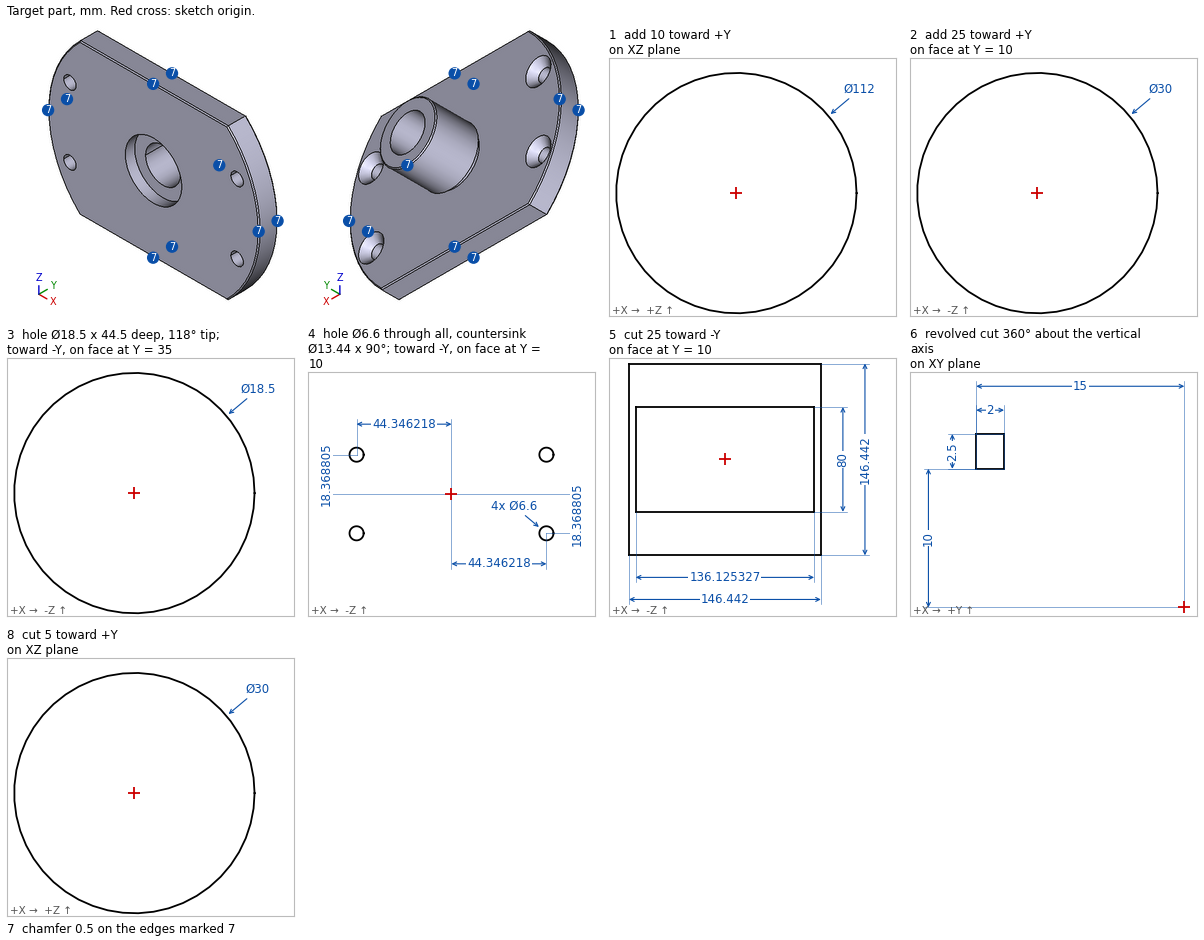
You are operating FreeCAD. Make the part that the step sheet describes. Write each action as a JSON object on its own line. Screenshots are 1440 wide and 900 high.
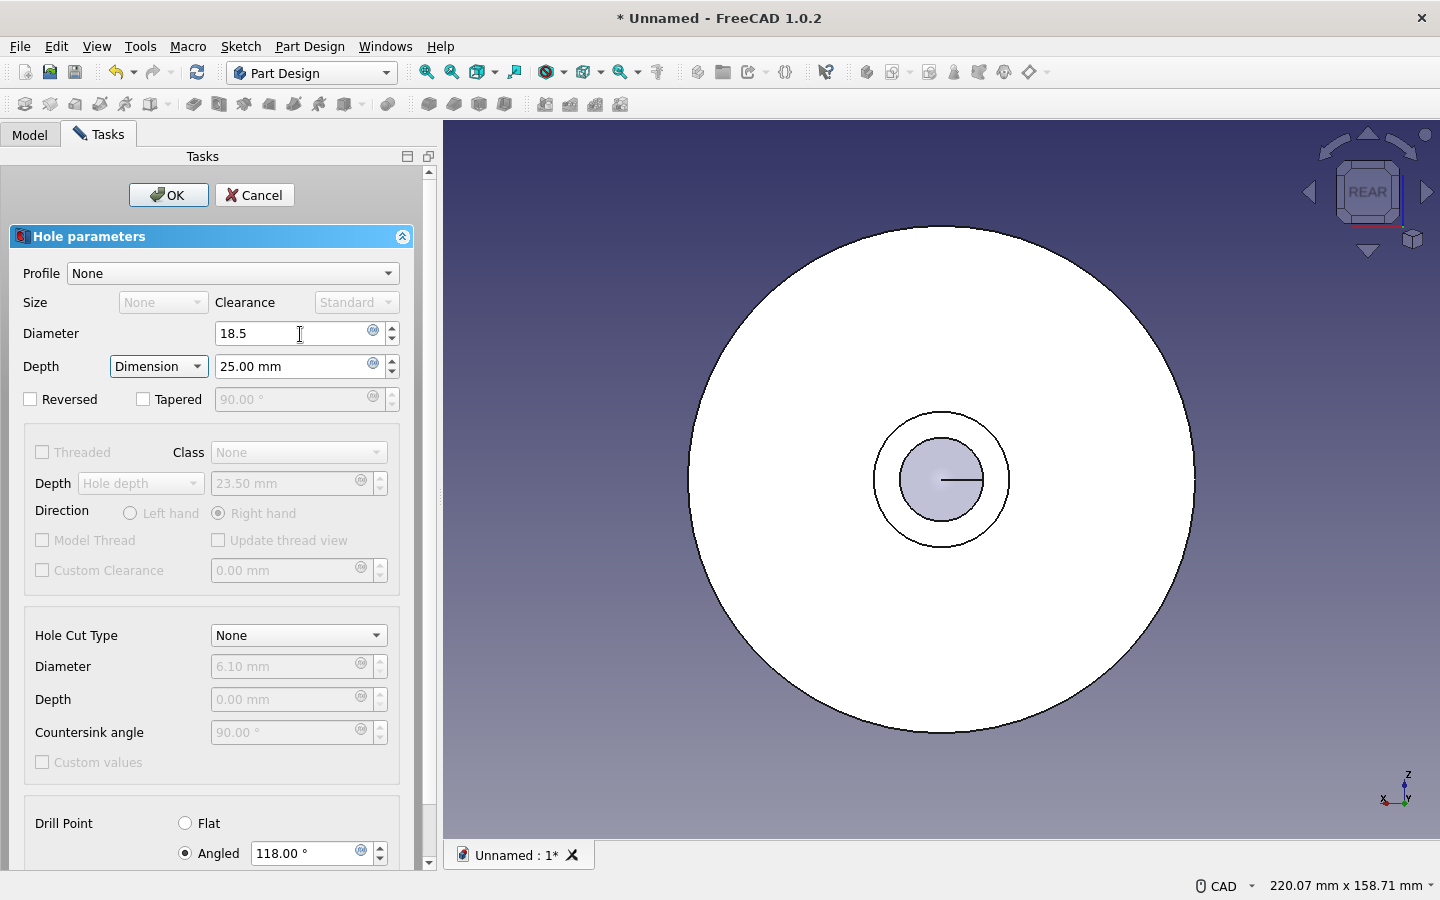
{"action": "triple_click", "coordinate": [300, 366]}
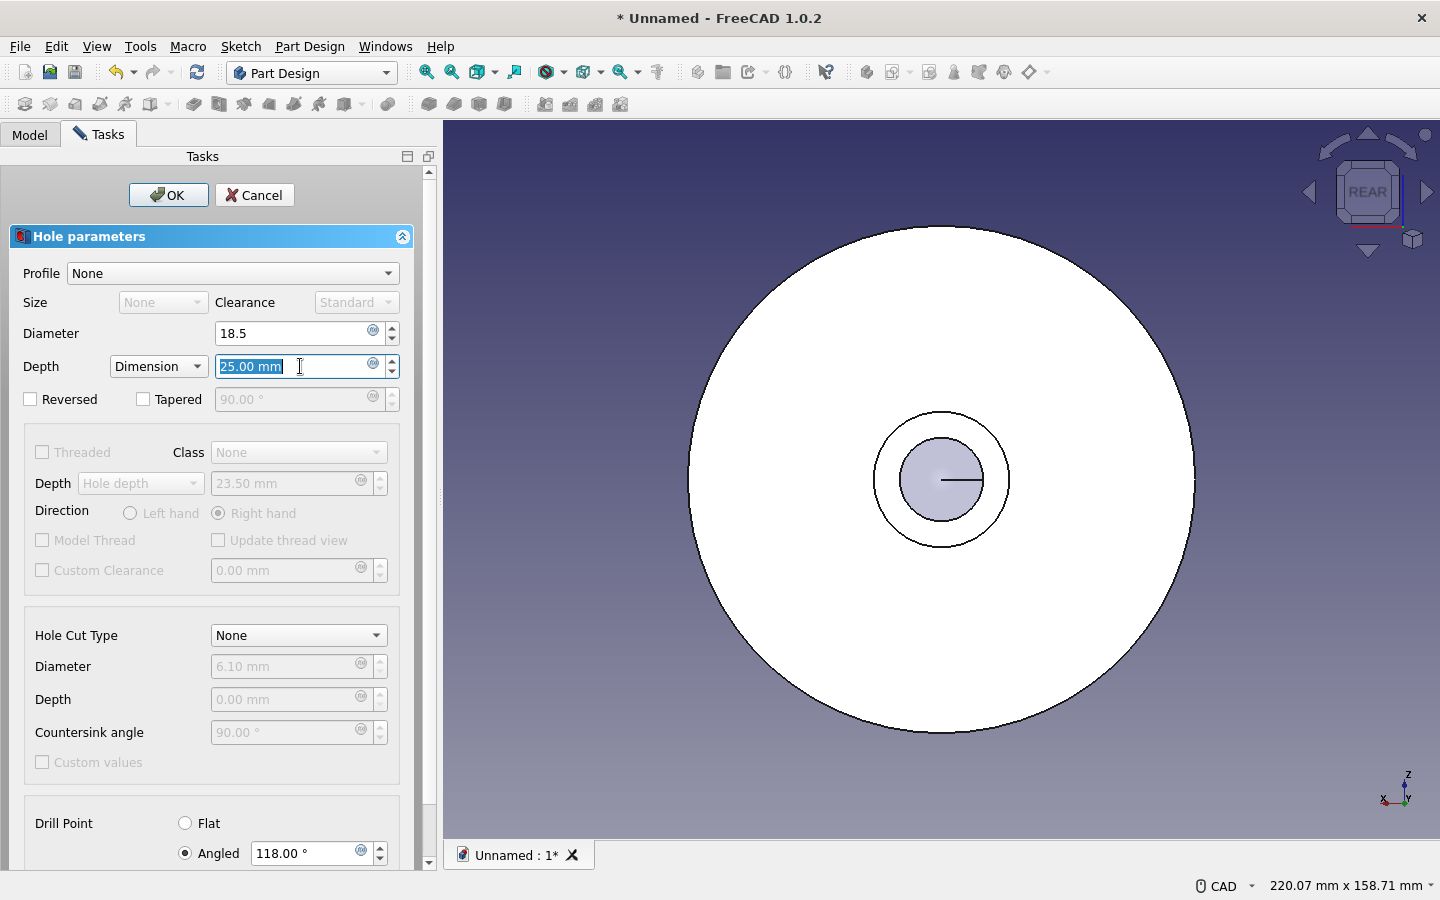
{"action": "type", "text": "44.5"}
{"action": "key", "text": "Tab"}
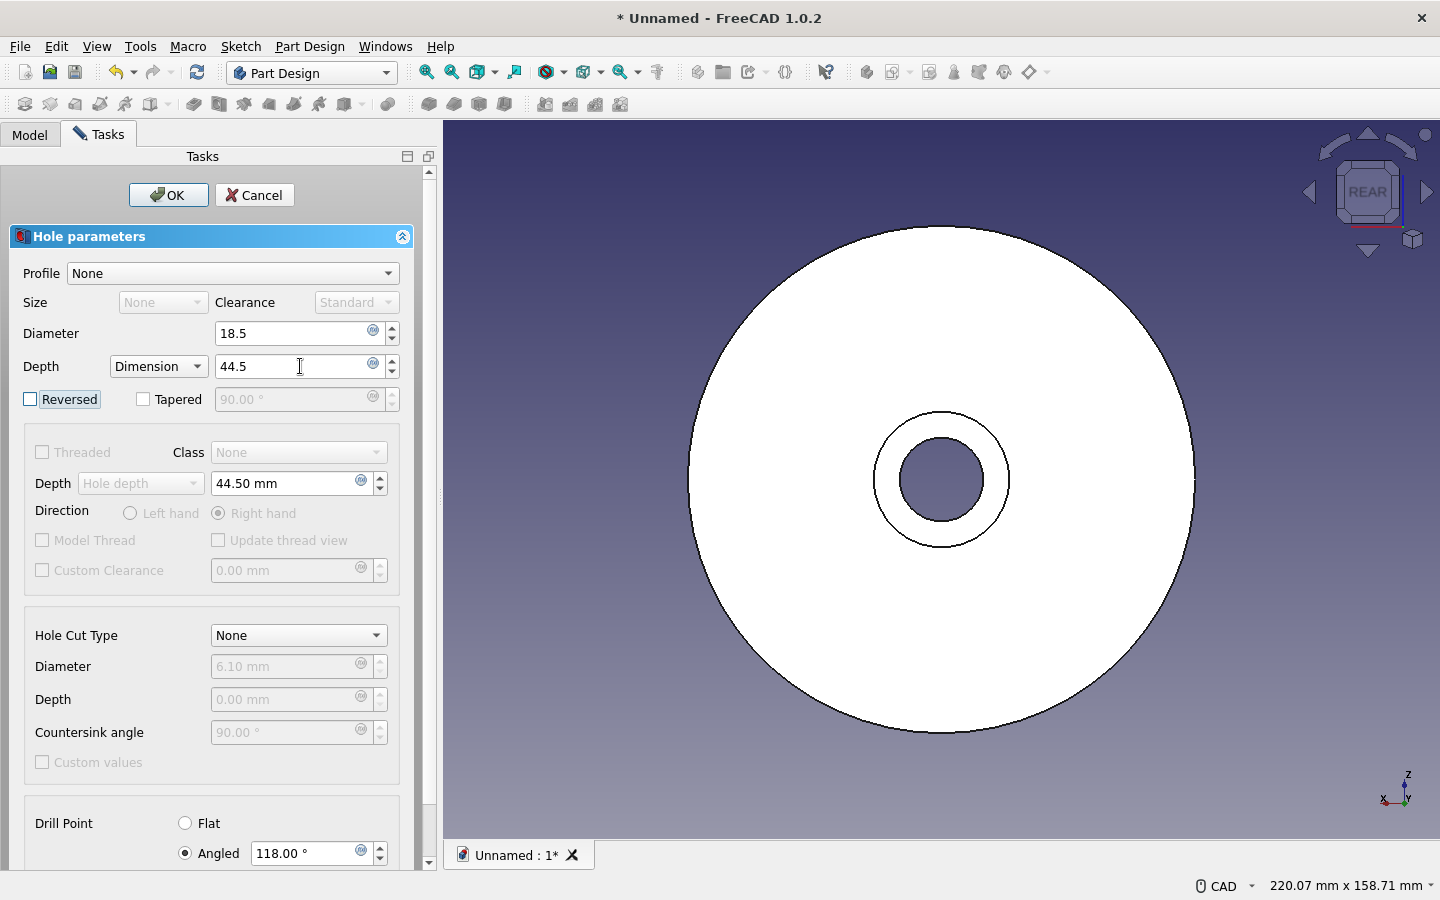
{"action": "left_click", "coordinate": [169, 195]}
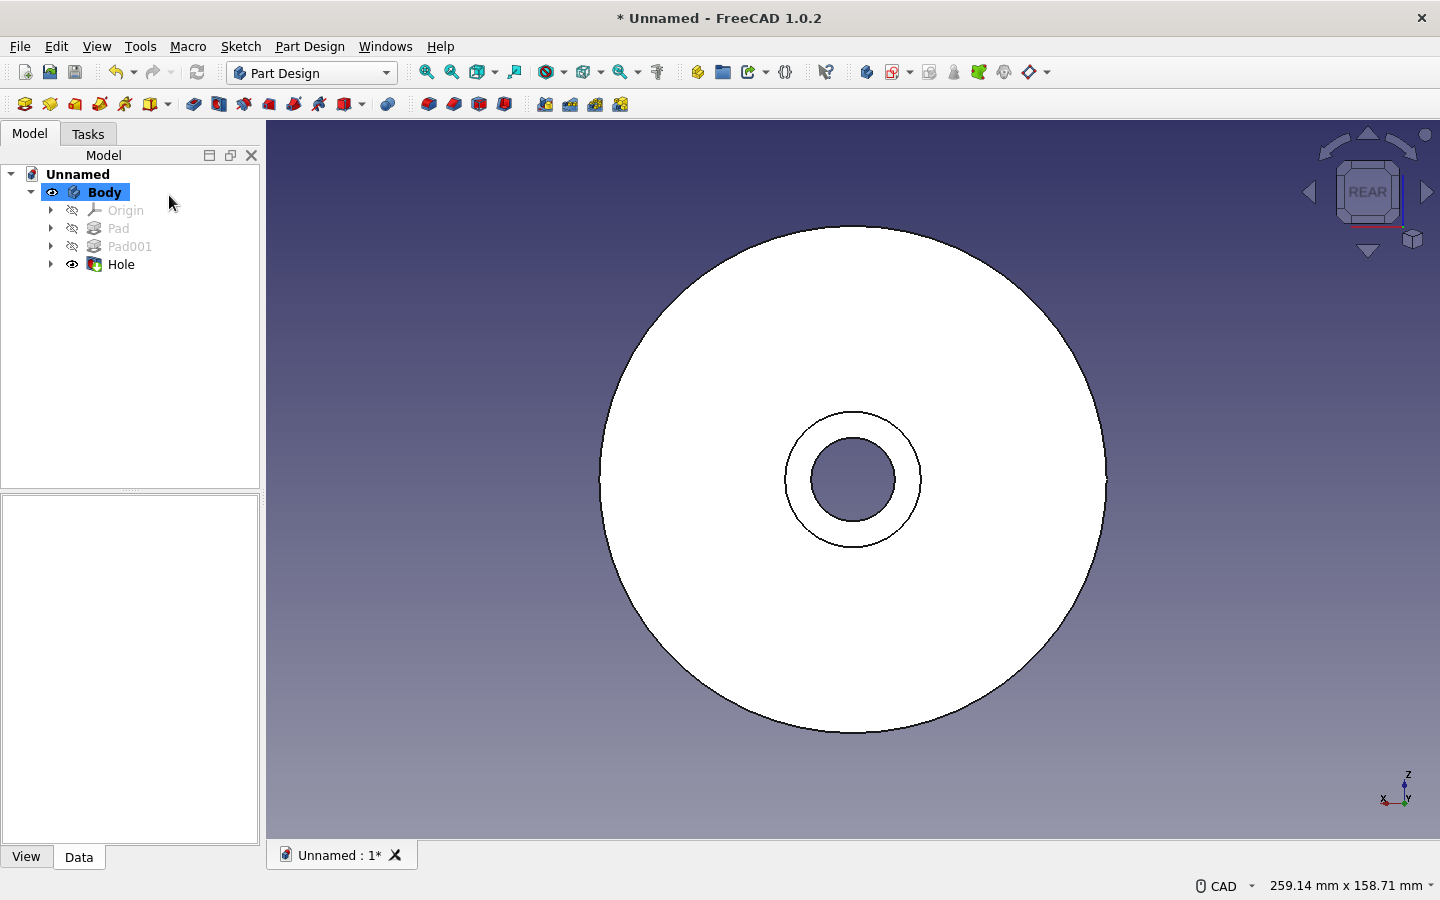
{"action": "left_click", "coordinate": [781, 334]}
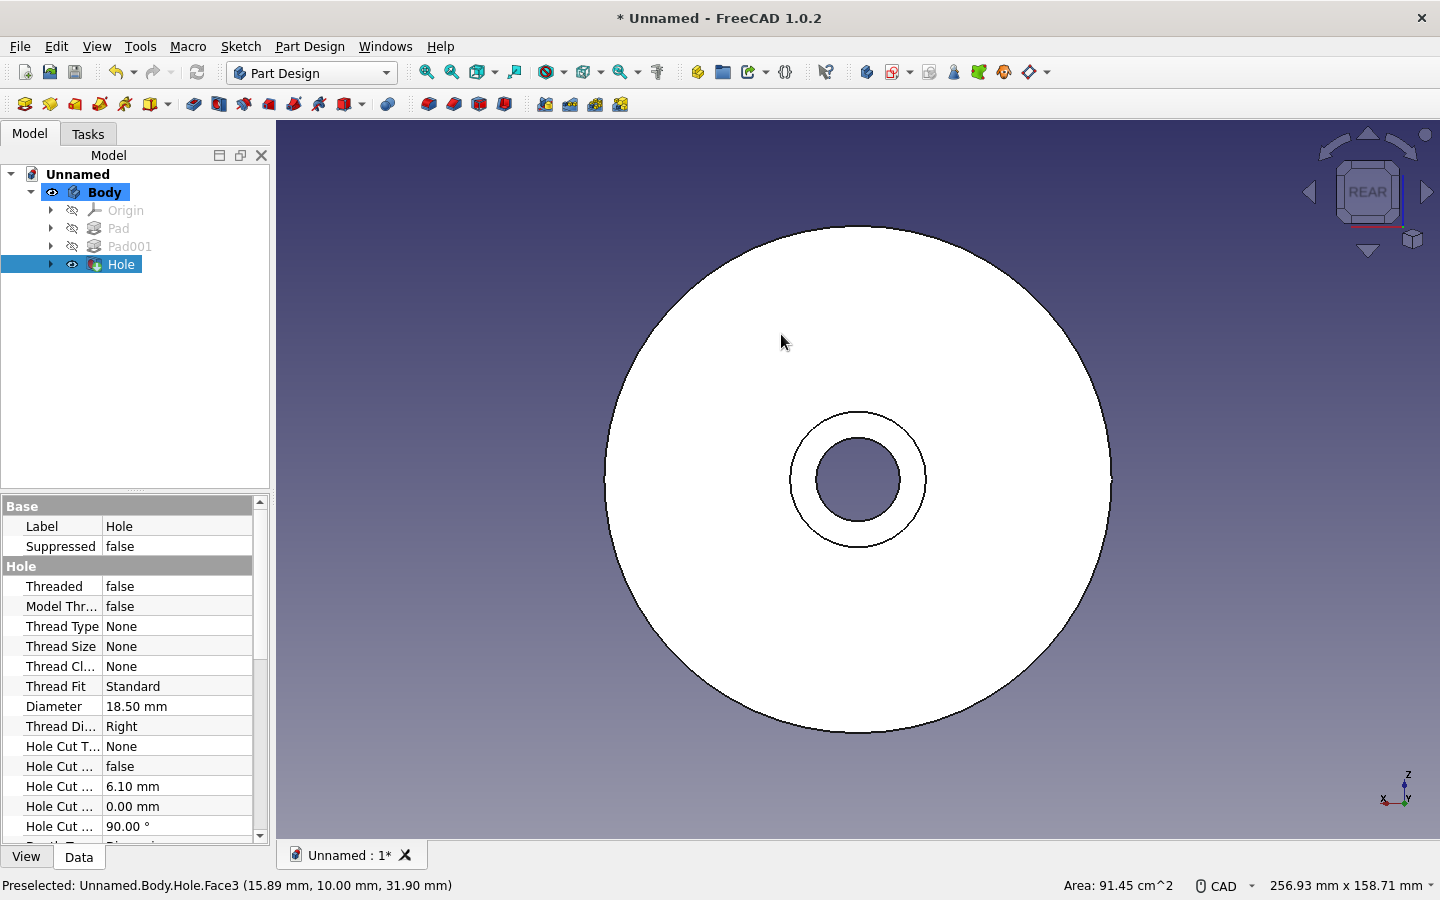
{"action": "left_click", "coordinate": [892, 72]}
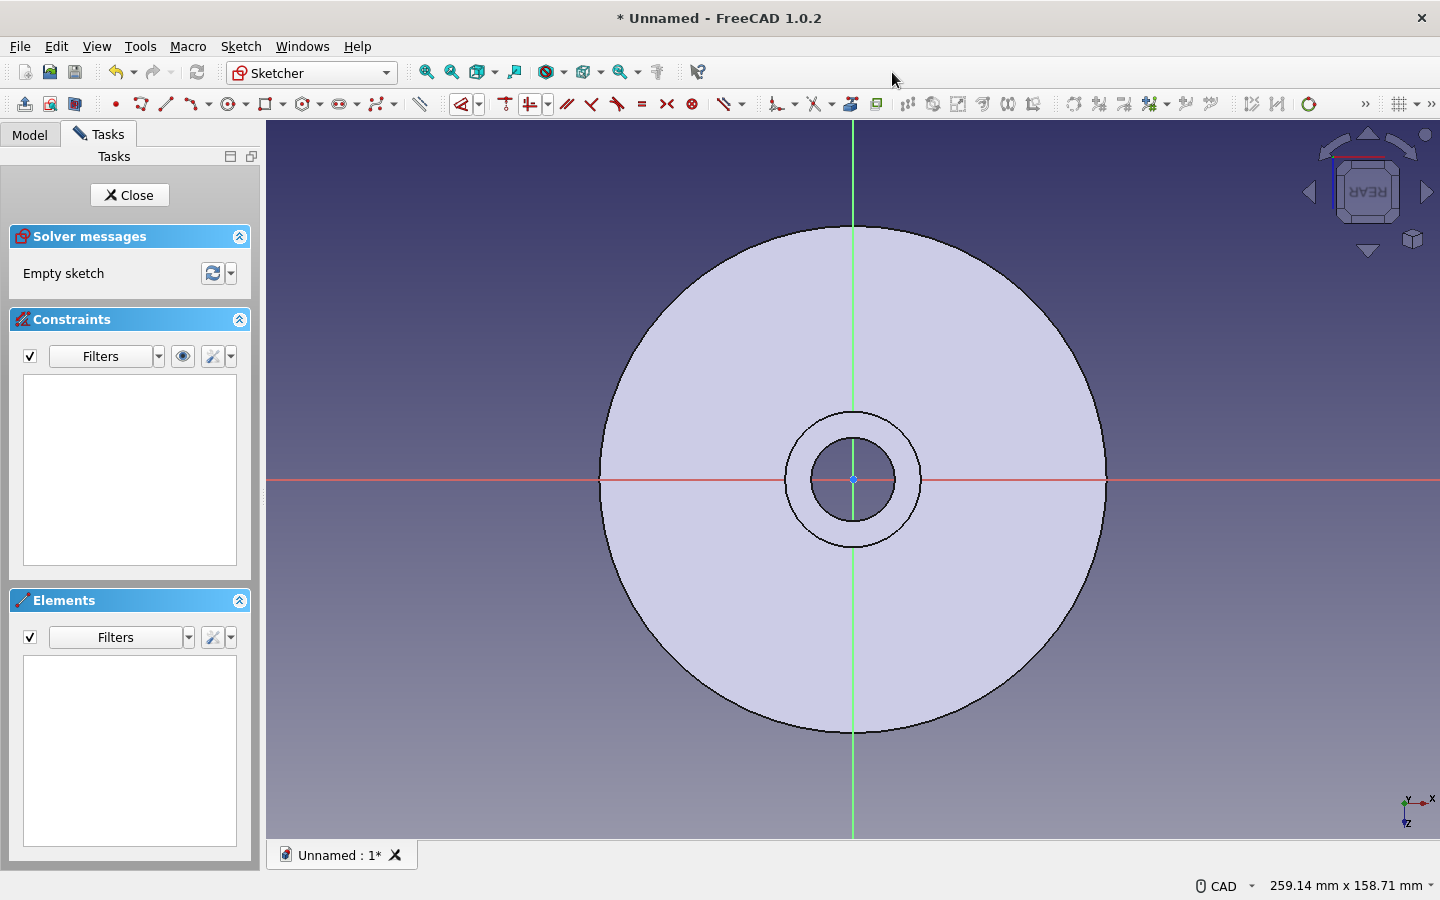
{"action": "left_click", "coordinate": [75, 104]}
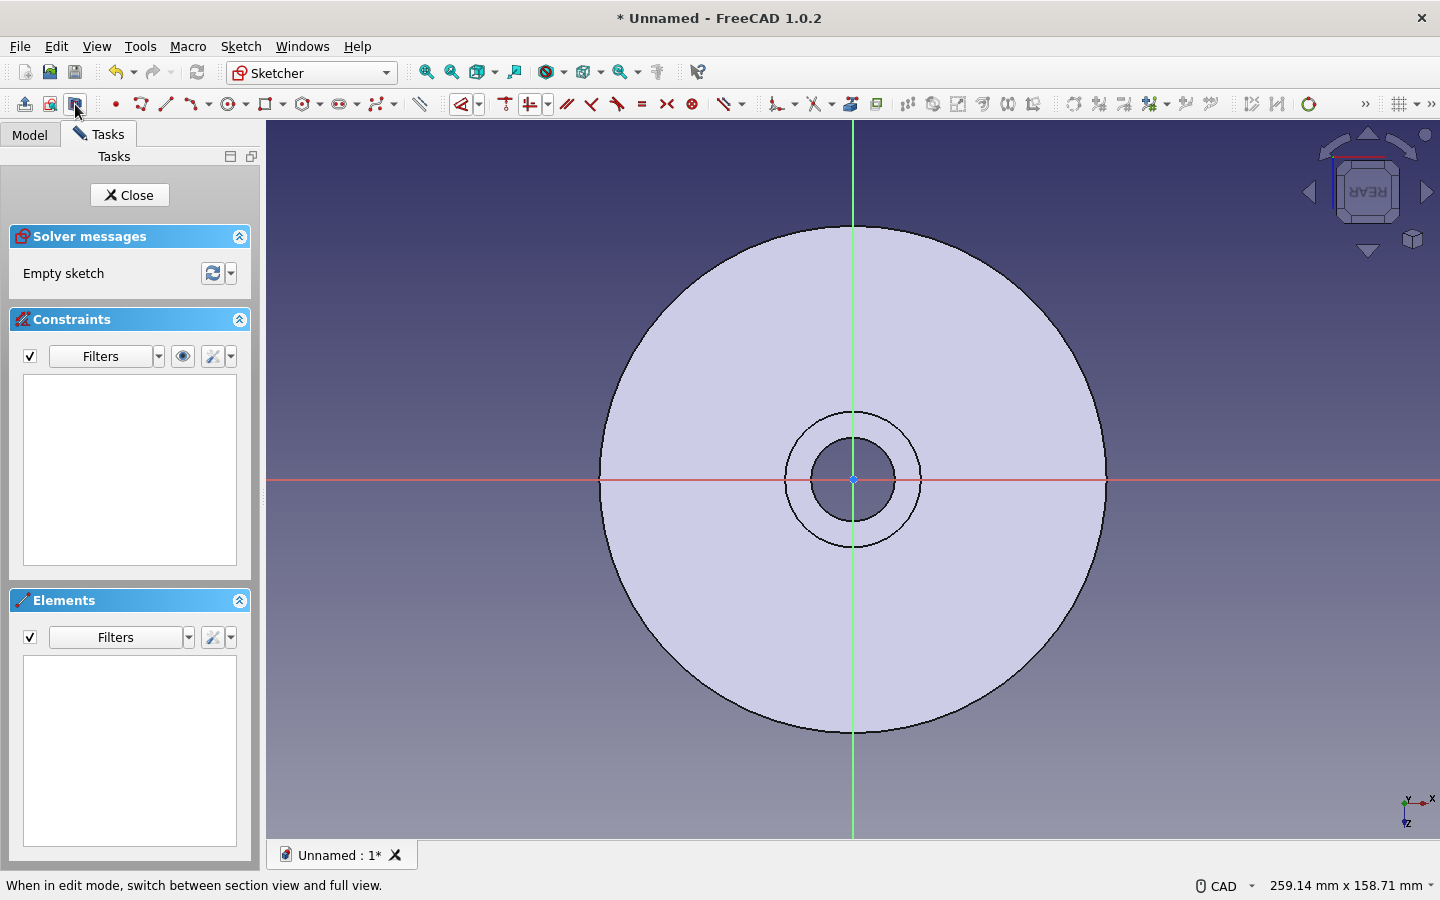
{"action": "scroll", "coordinate": [992, 479], "scroll_direction": "up", "scroll_amount": 2}